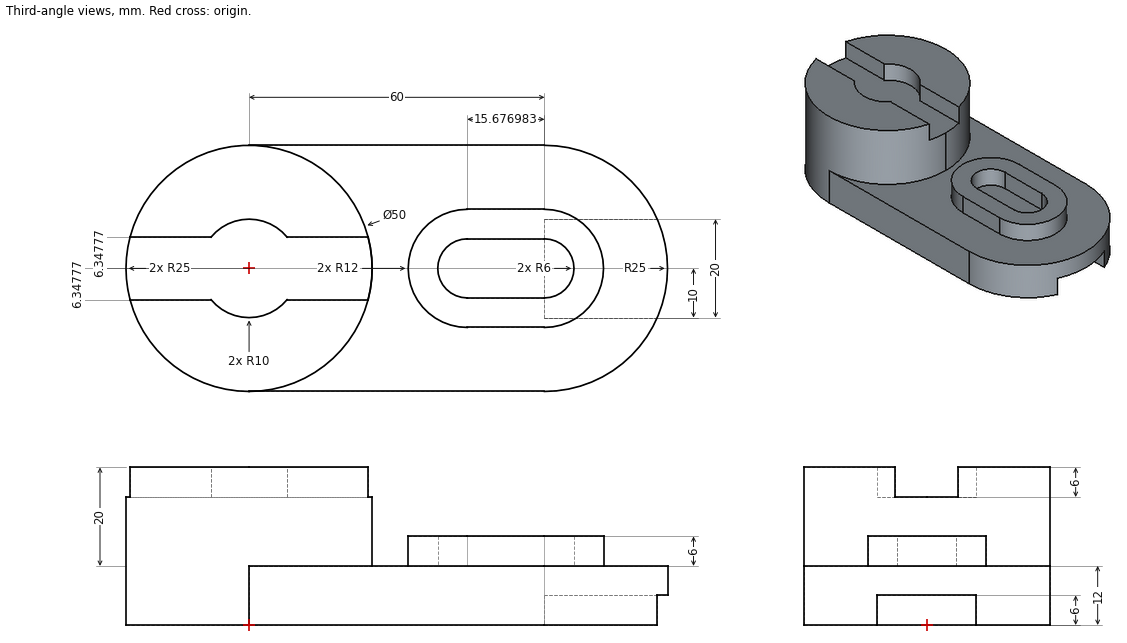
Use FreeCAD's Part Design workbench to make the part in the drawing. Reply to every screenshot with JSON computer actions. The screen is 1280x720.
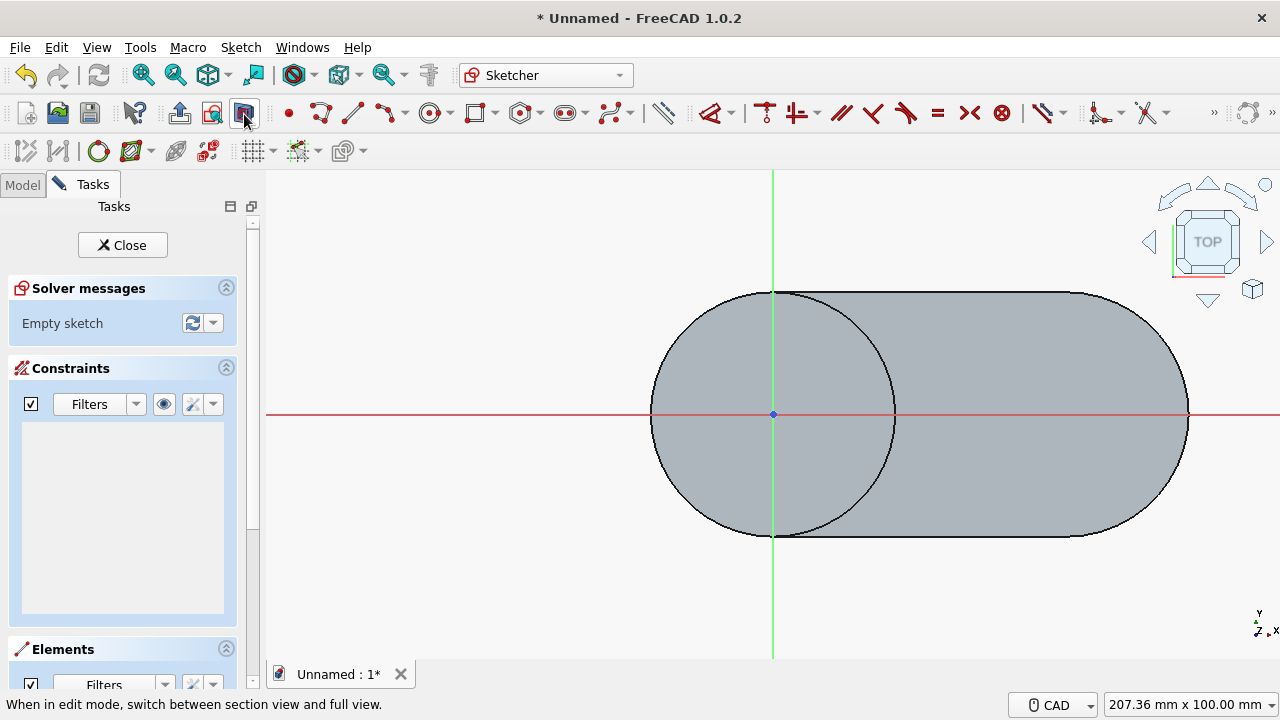
{"action": "scroll", "coordinate": [294, 415], "scroll_direction": "down", "scroll_amount": 1}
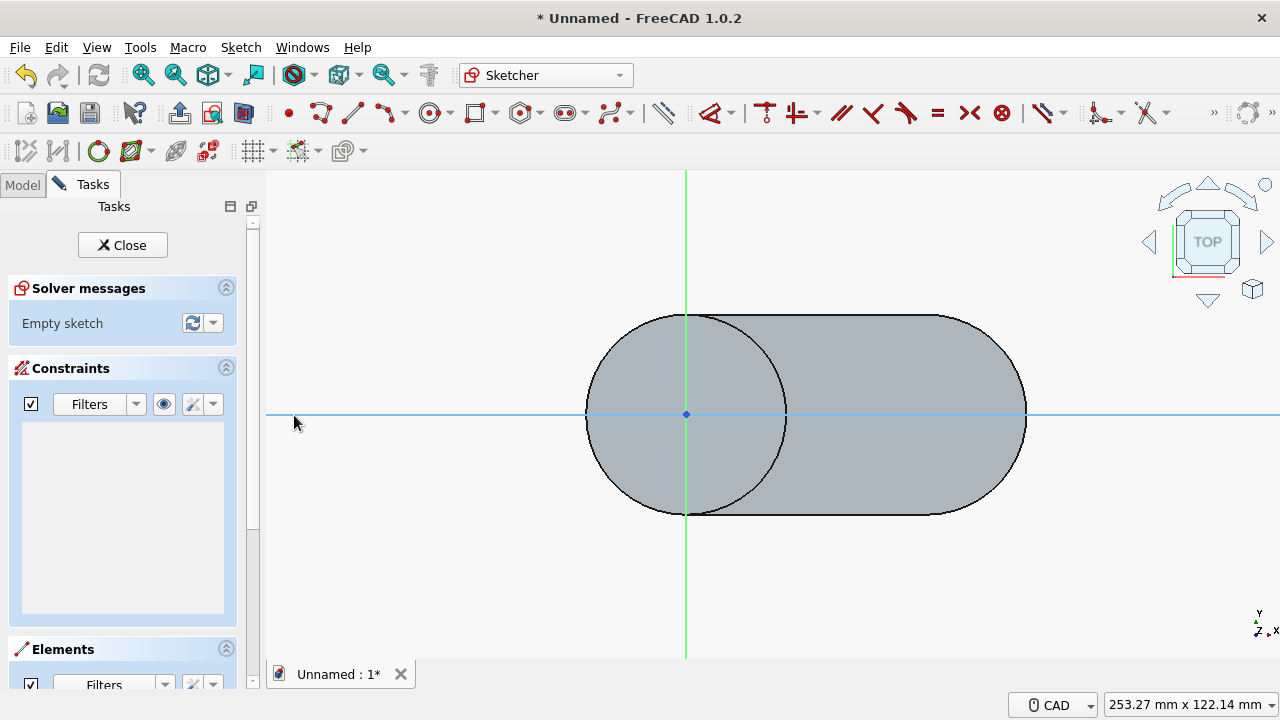
{"action": "scroll", "coordinate": [983, 415], "scroll_direction": "up", "scroll_amount": 3}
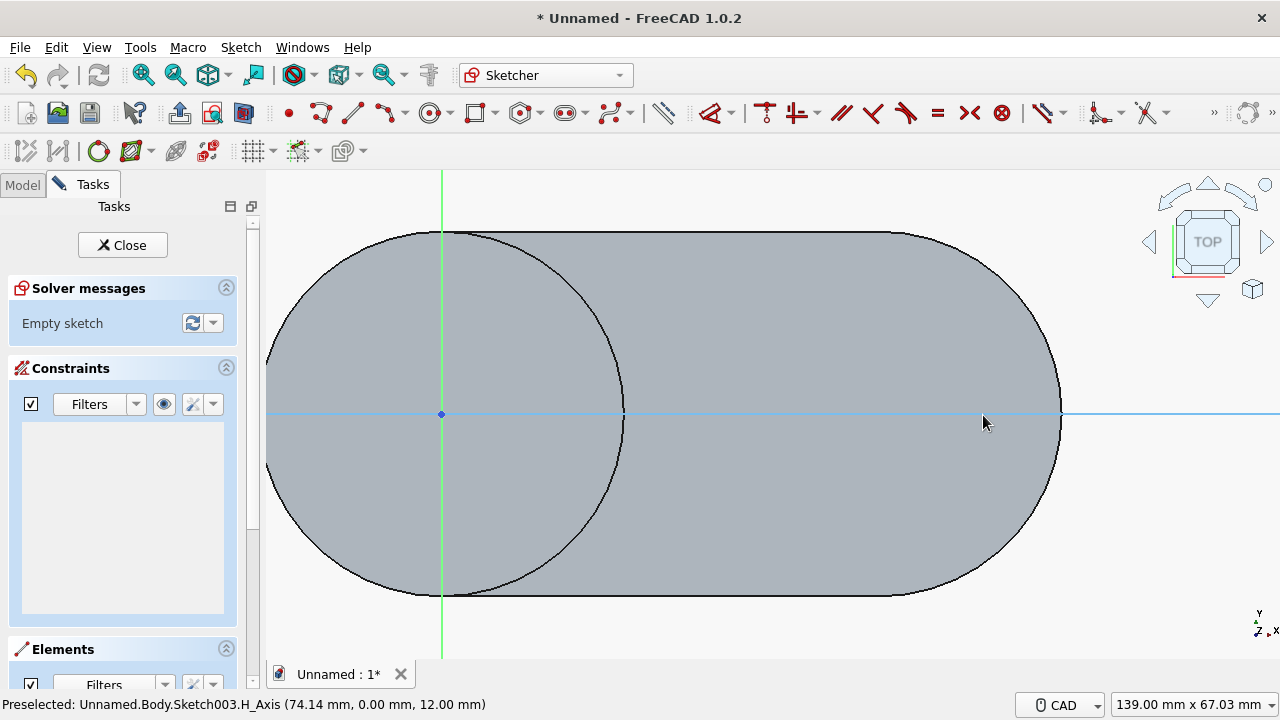
{"action": "left_click", "coordinate": [566, 114]}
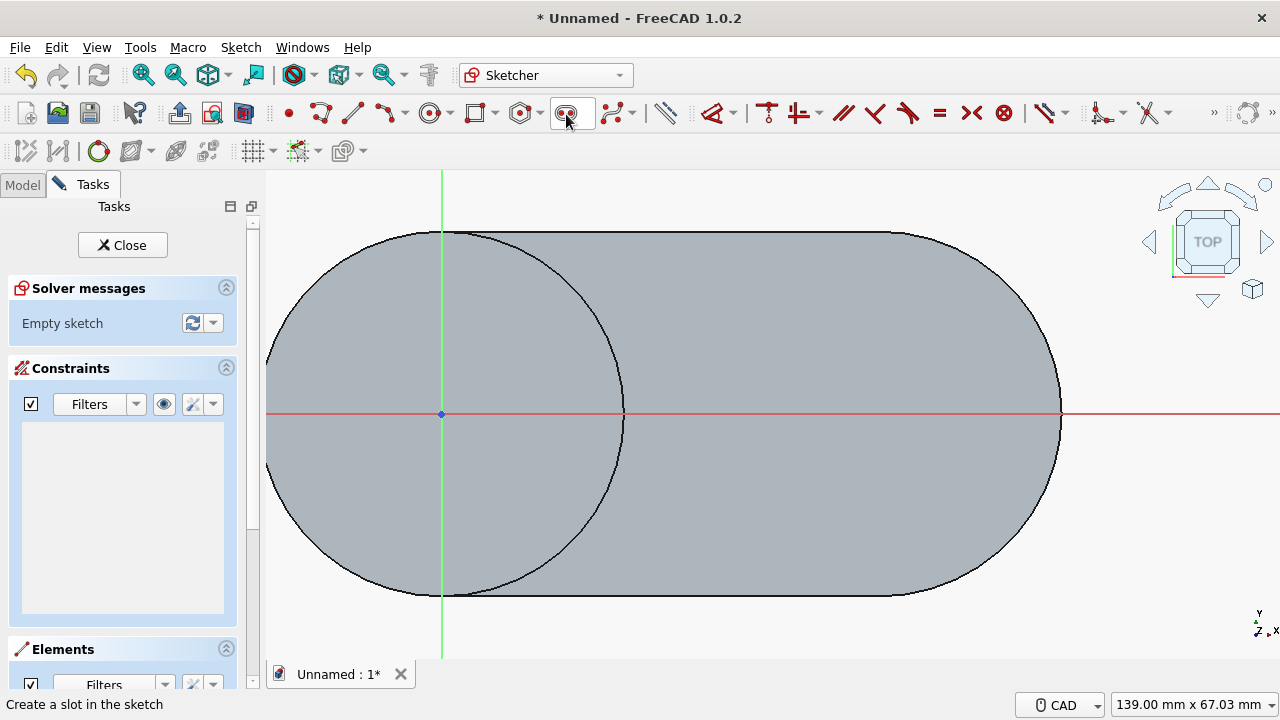
{"action": "left_click", "coordinate": [765, 414]}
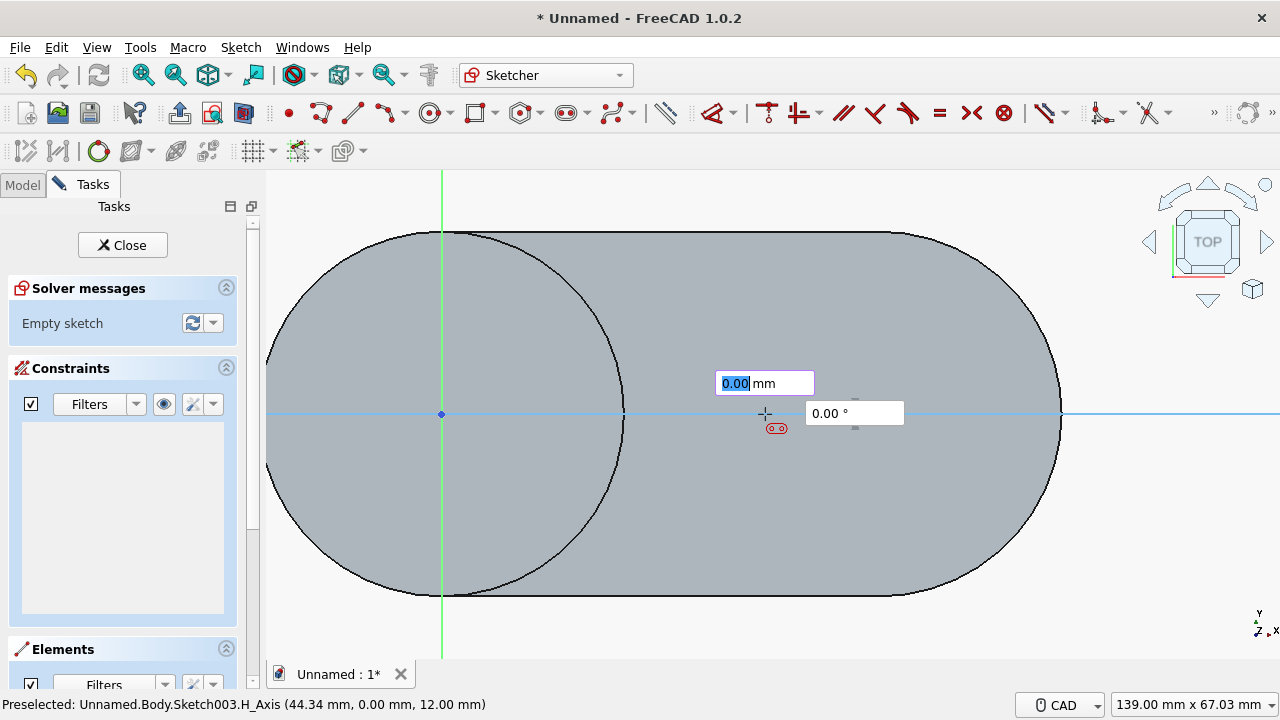
{"action": "left_click", "coordinate": [879, 405]}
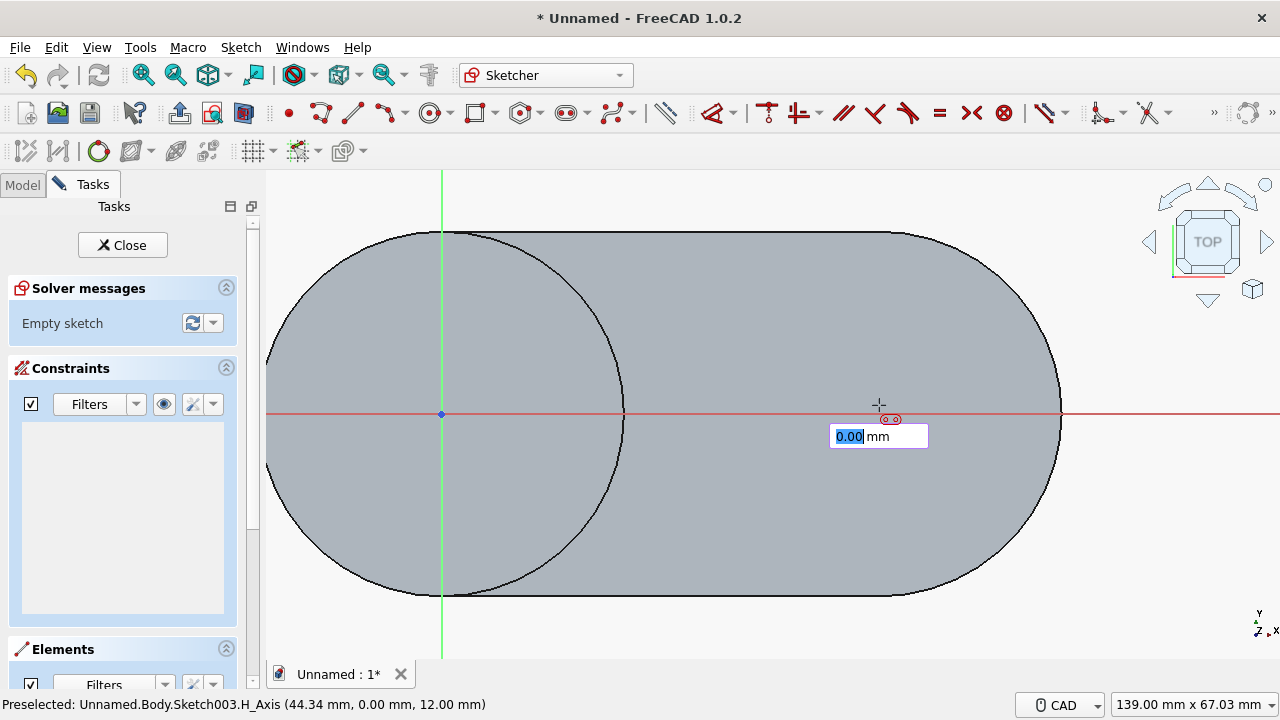
{"action": "left_click", "coordinate": [822, 326]}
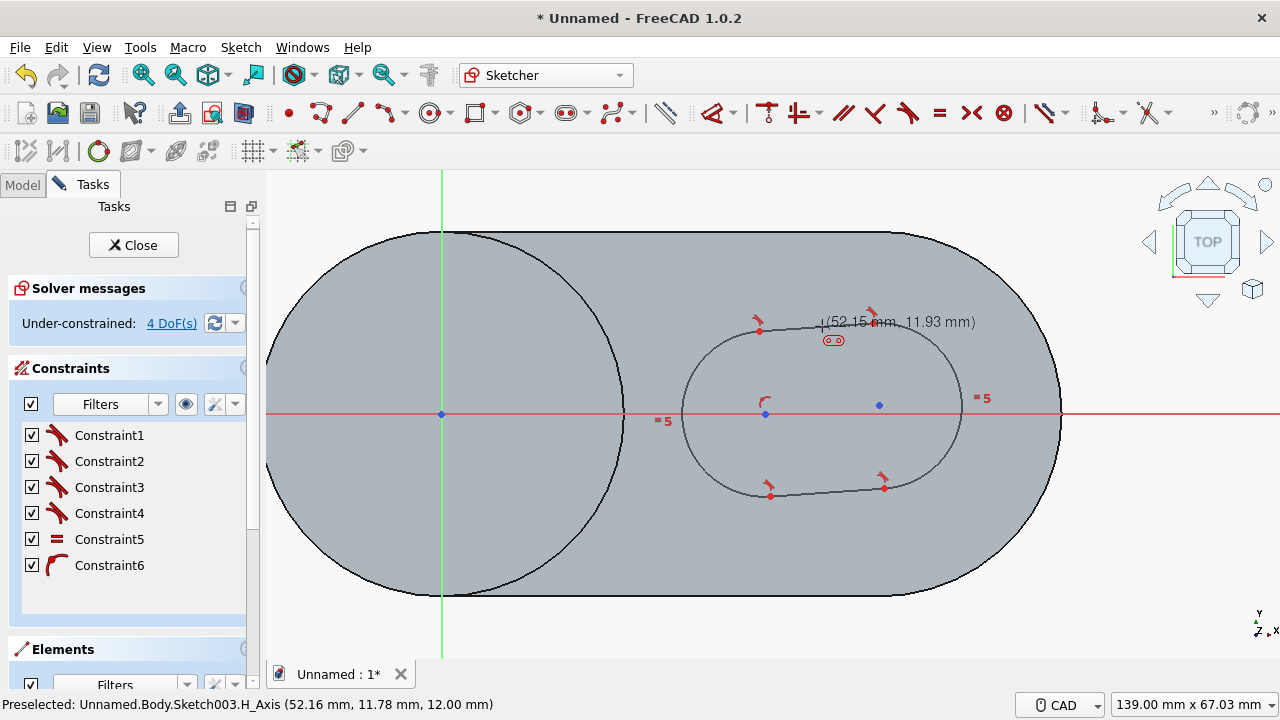
{"action": "left_click", "coordinate": [765, 414]}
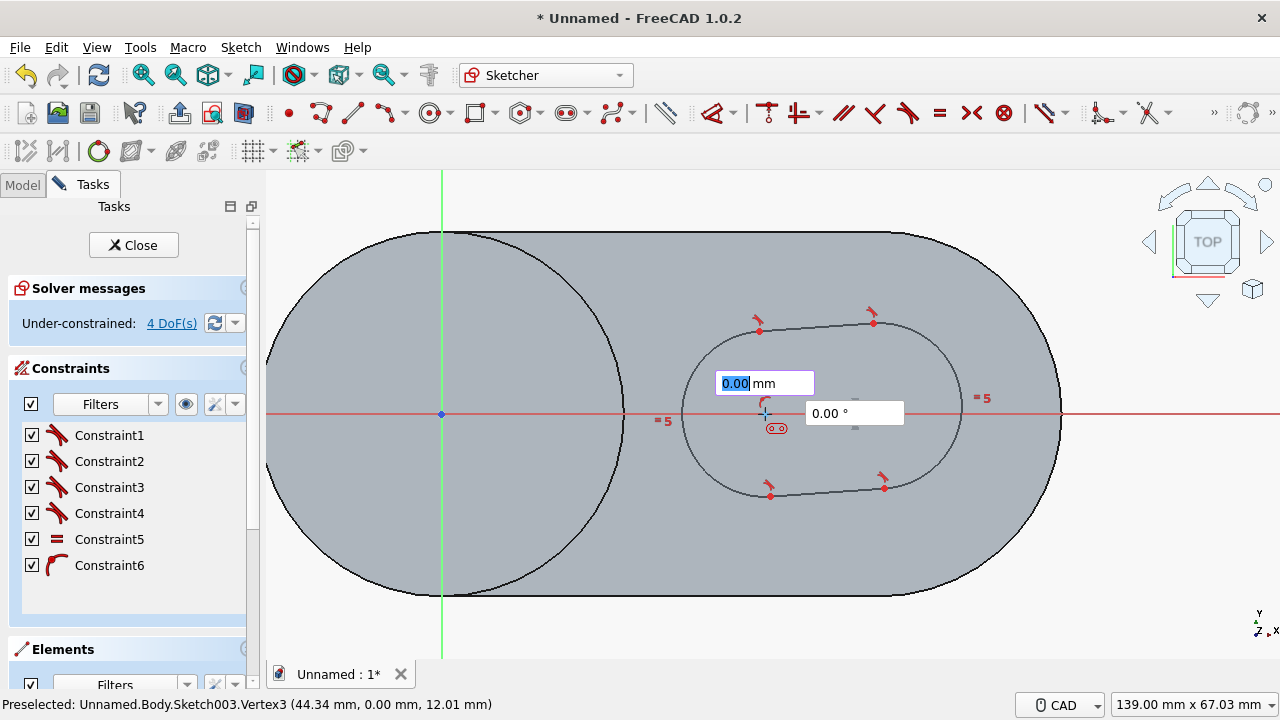
{"action": "left_click", "coordinate": [879, 406]}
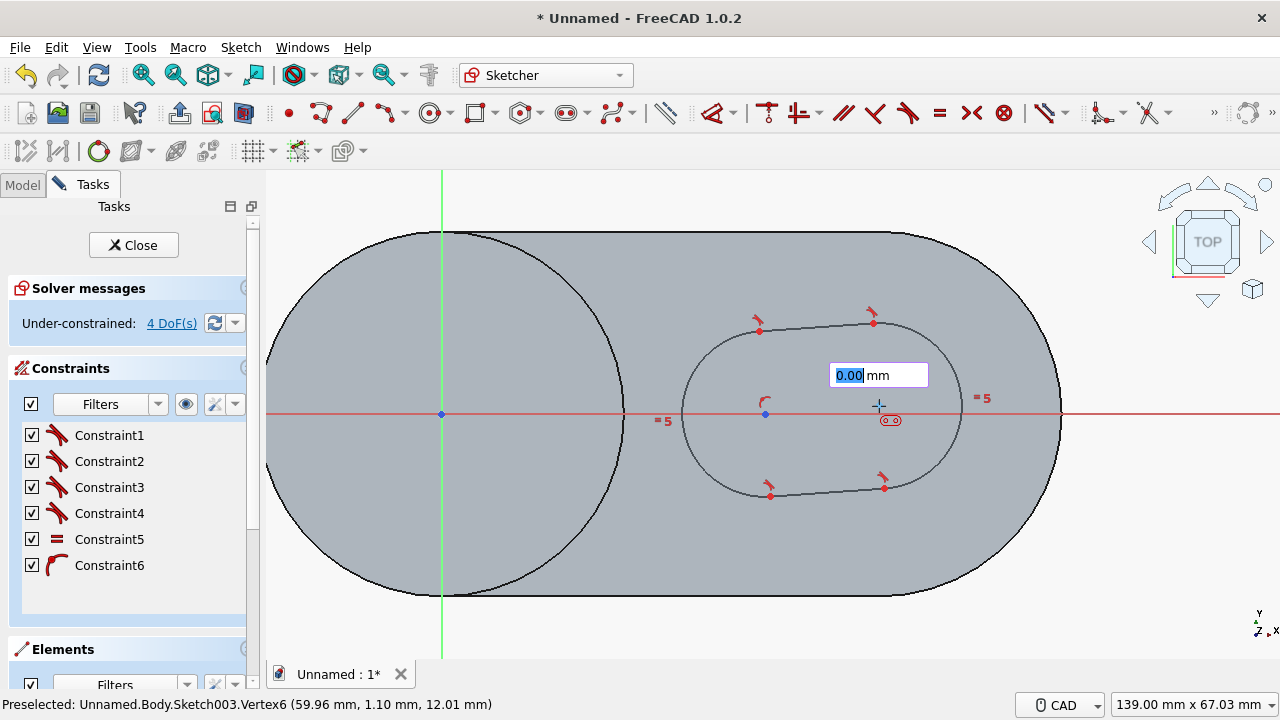
{"action": "left_click", "coordinate": [822, 370]}
{"action": "key", "text": "Escape"}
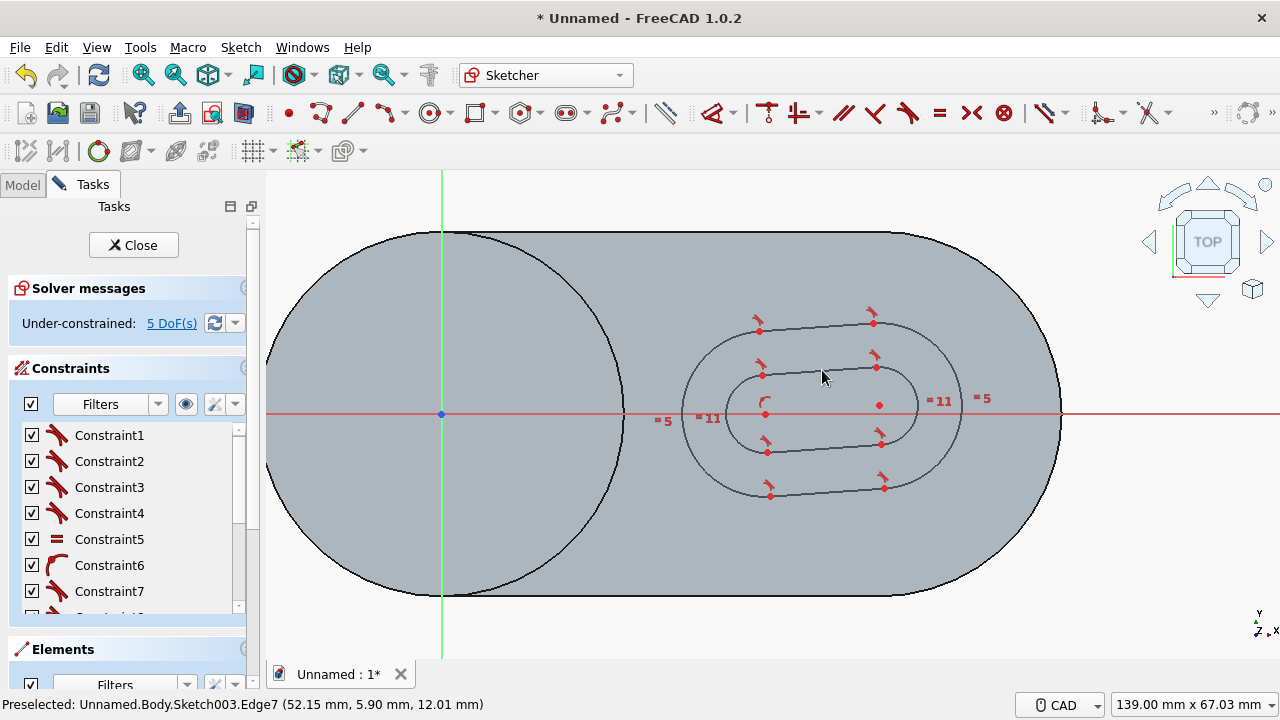
{"action": "left_click", "coordinate": [793, 329]}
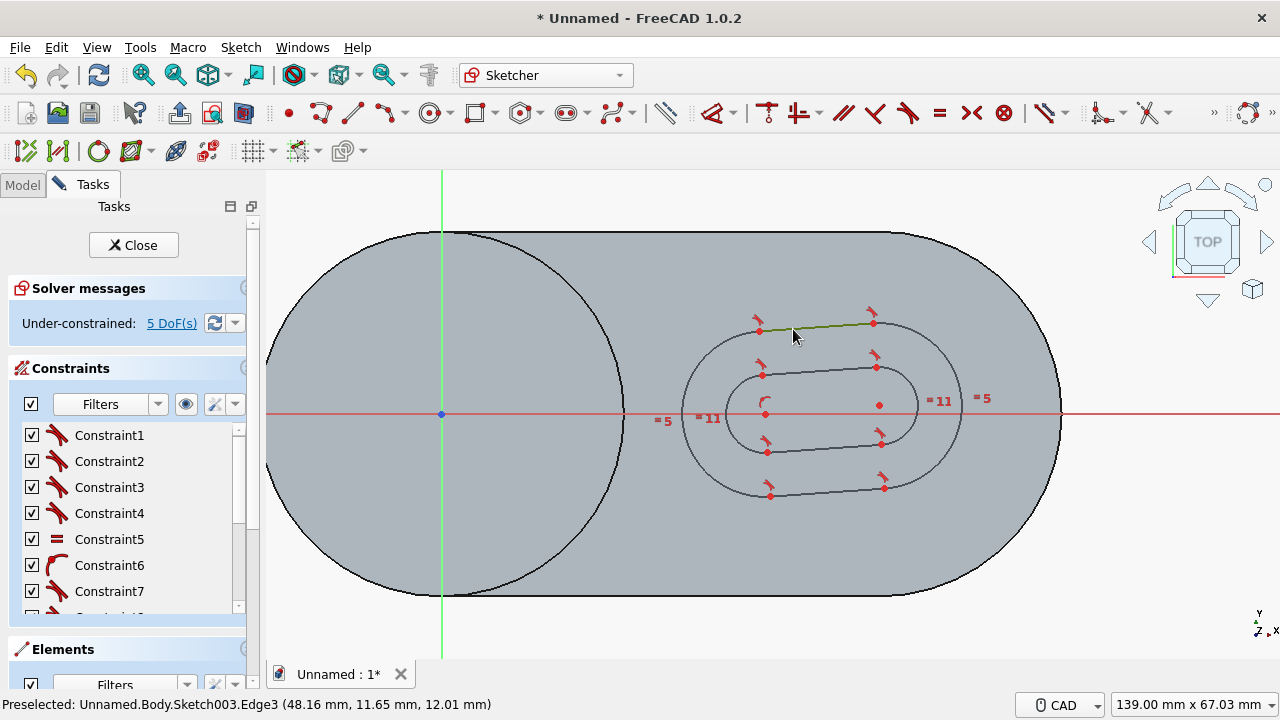
{"action": "key", "text": "h"}